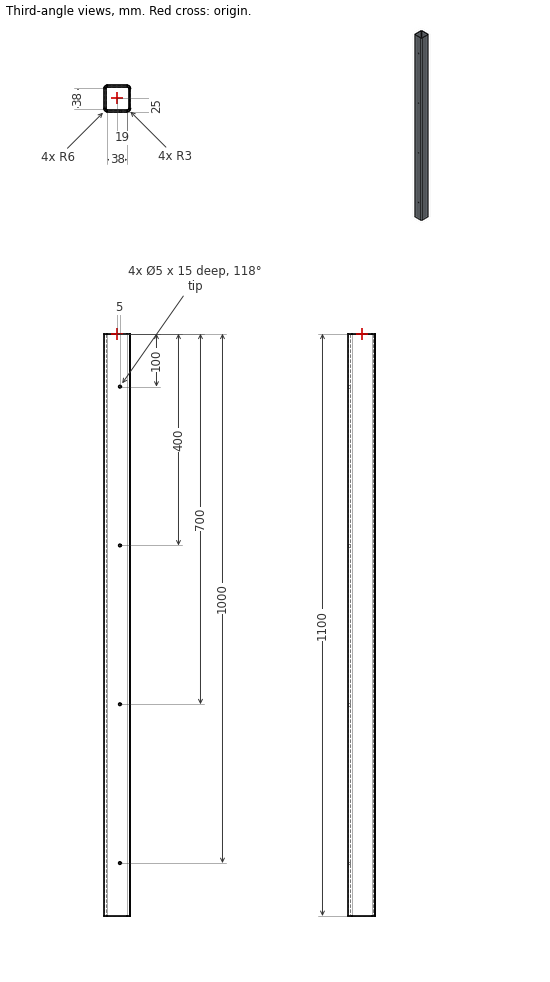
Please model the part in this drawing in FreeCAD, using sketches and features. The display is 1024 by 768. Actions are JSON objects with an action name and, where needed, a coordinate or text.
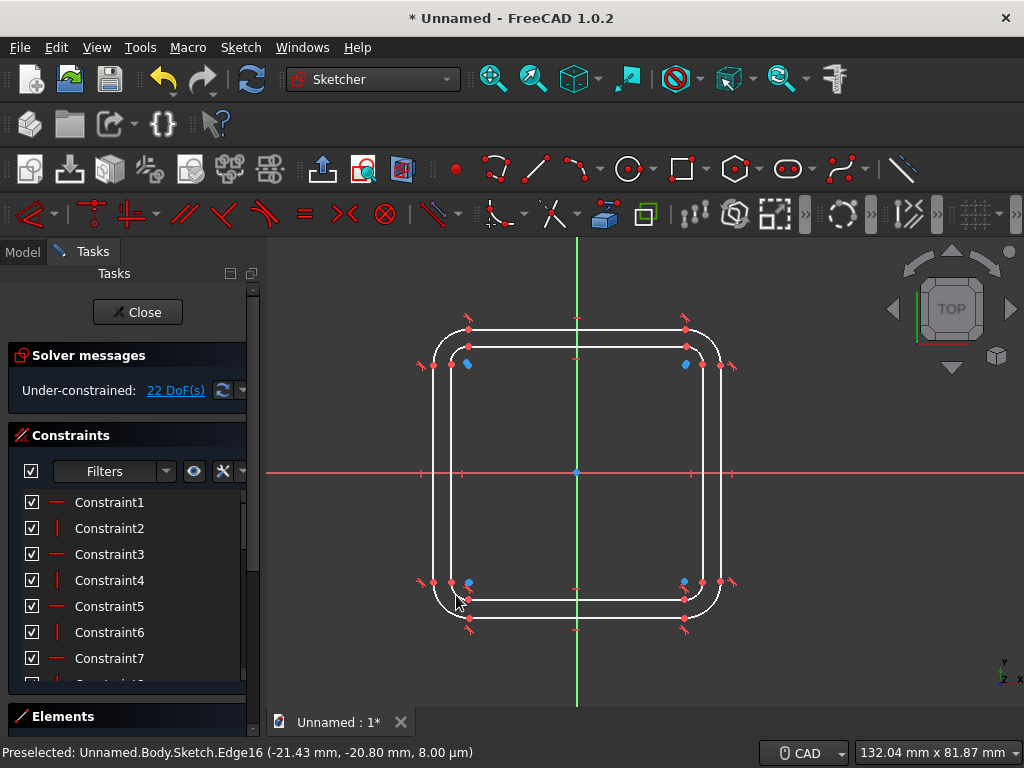
{"action": "left_click", "coordinate": [703, 518]}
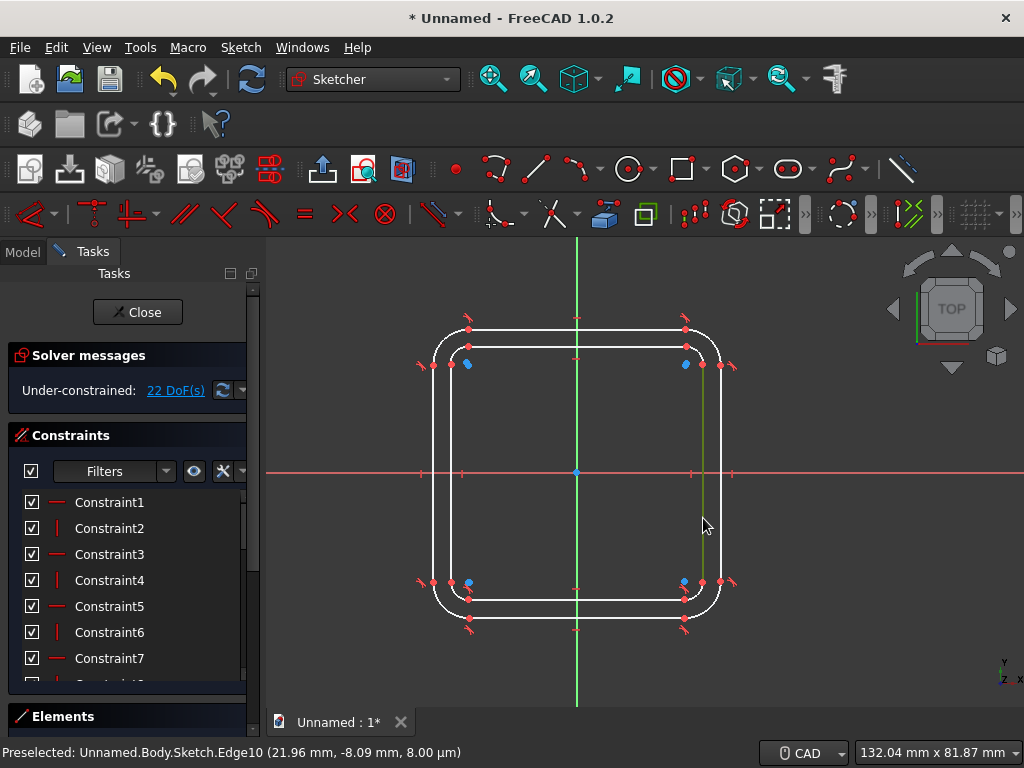
{"action": "left_click", "coordinate": [697, 595]}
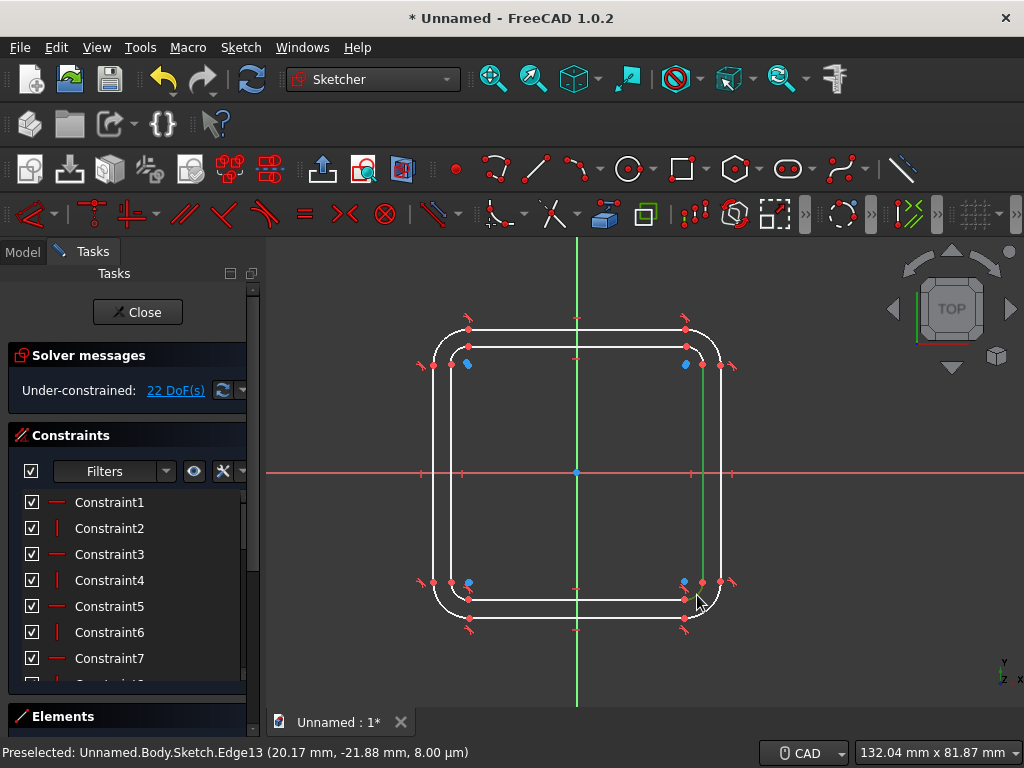
{"action": "key", "text": "t"}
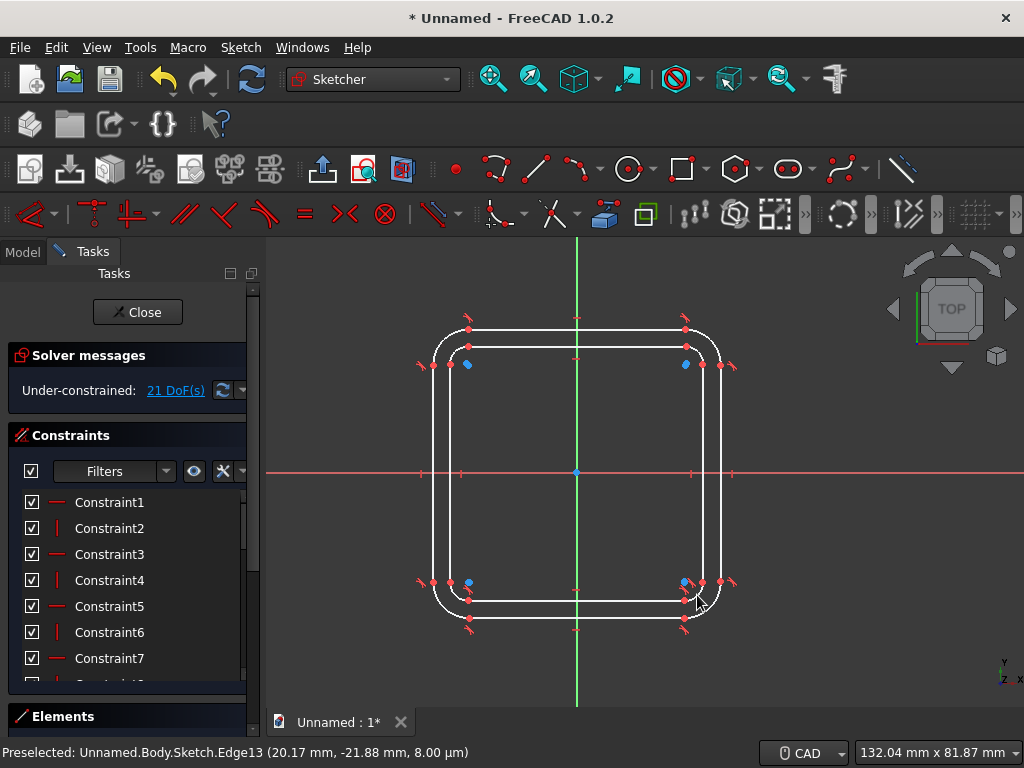
{"action": "left_click", "coordinate": [703, 517]}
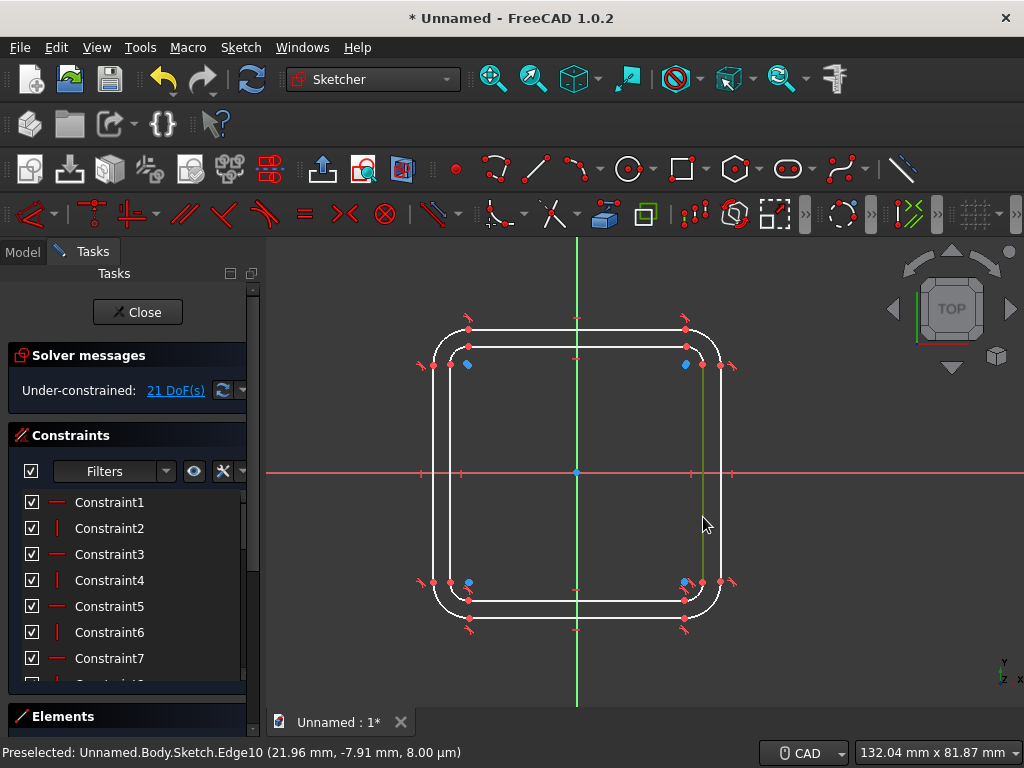
{"action": "left_click", "coordinate": [699, 352]}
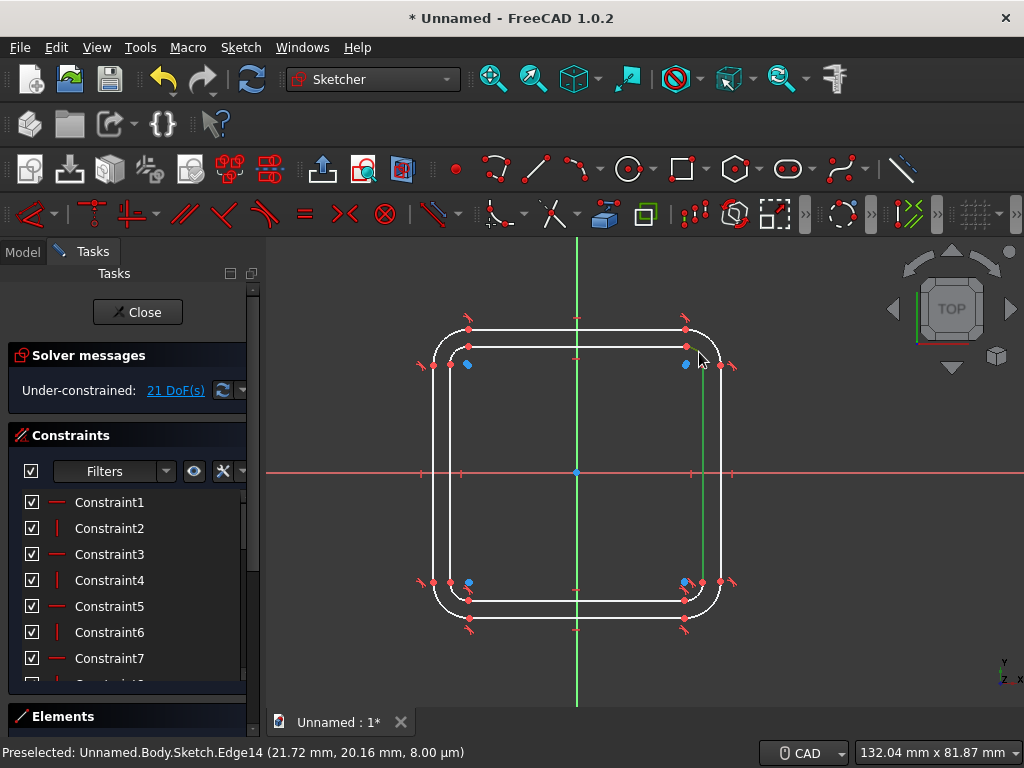
{"action": "key", "text": "t"}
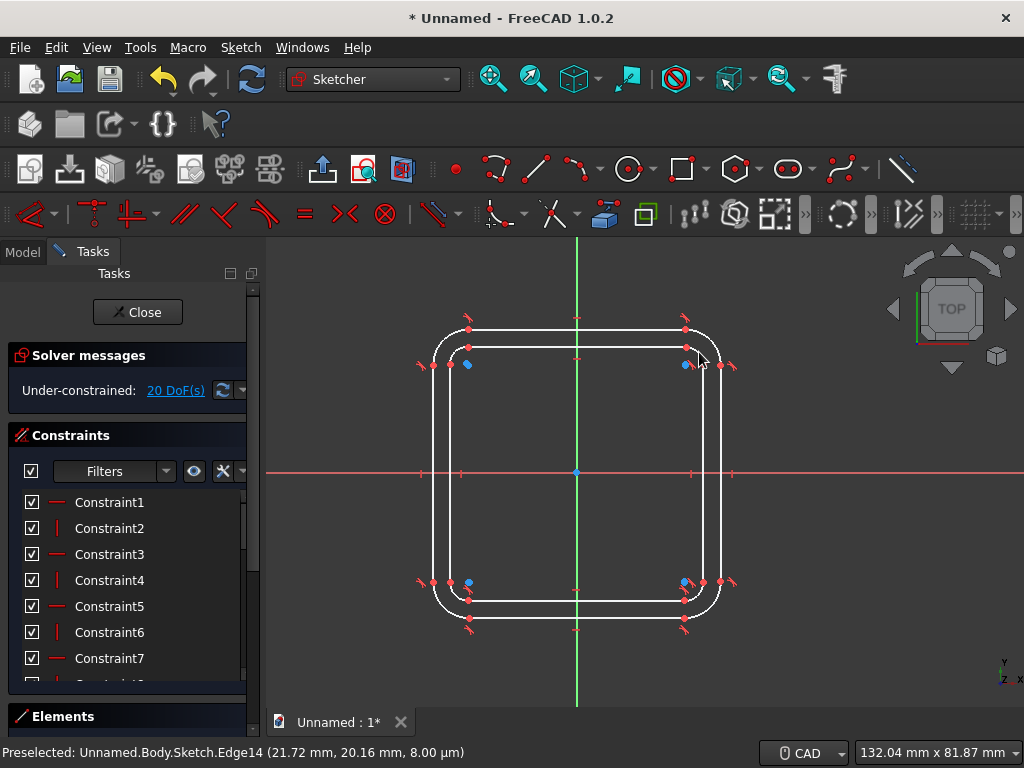
{"action": "left_click", "coordinate": [621, 347]}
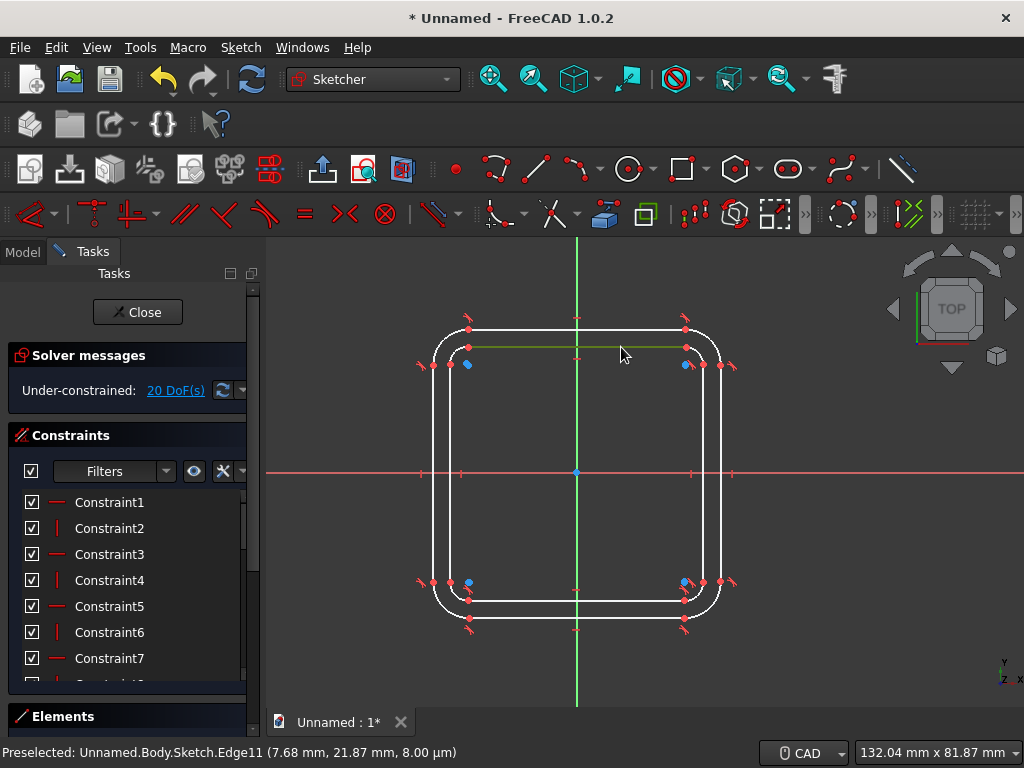
{"action": "left_click", "coordinate": [698, 353]}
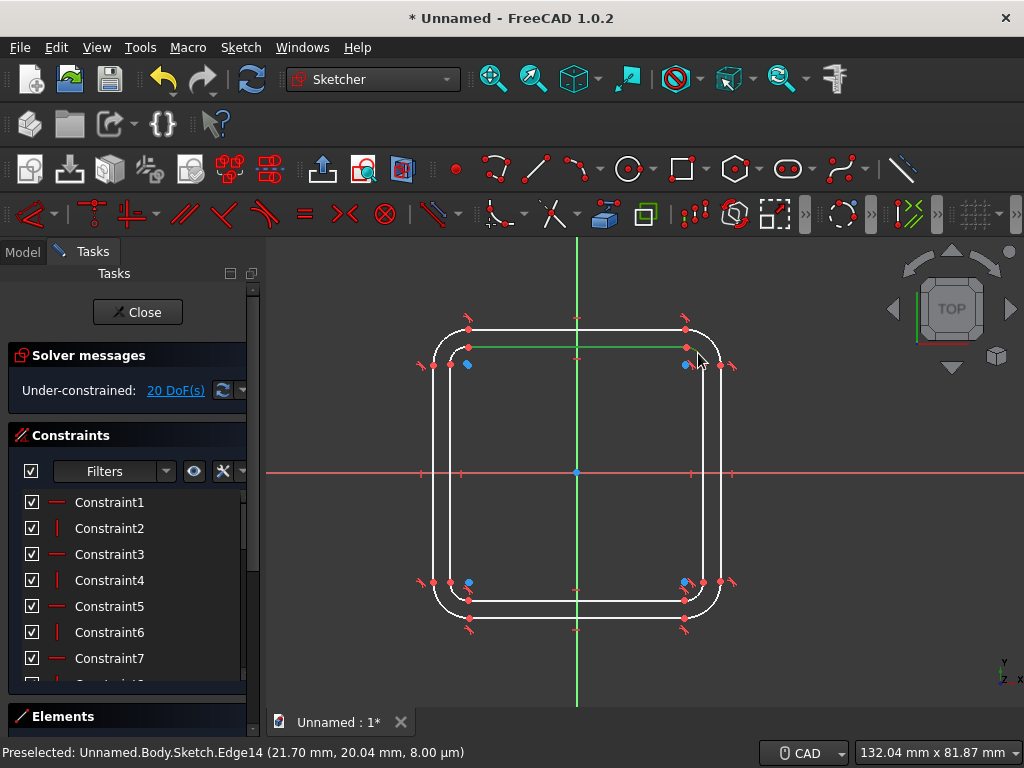
{"action": "key", "text": "t"}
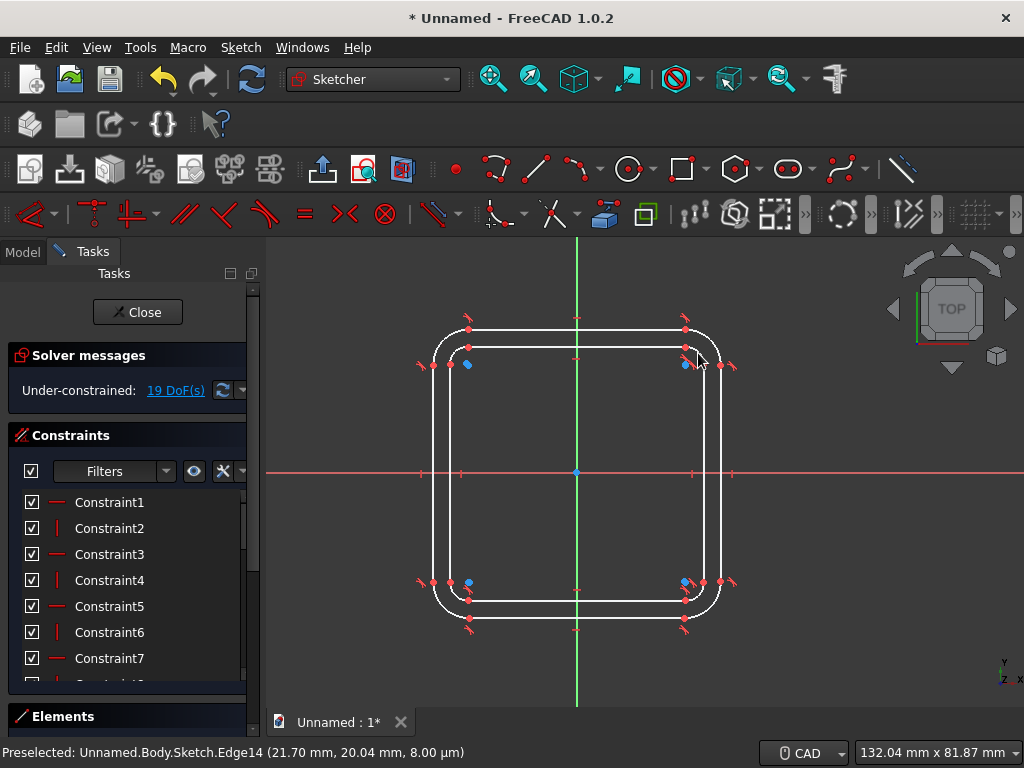
{"action": "left_click", "coordinate": [621, 347]}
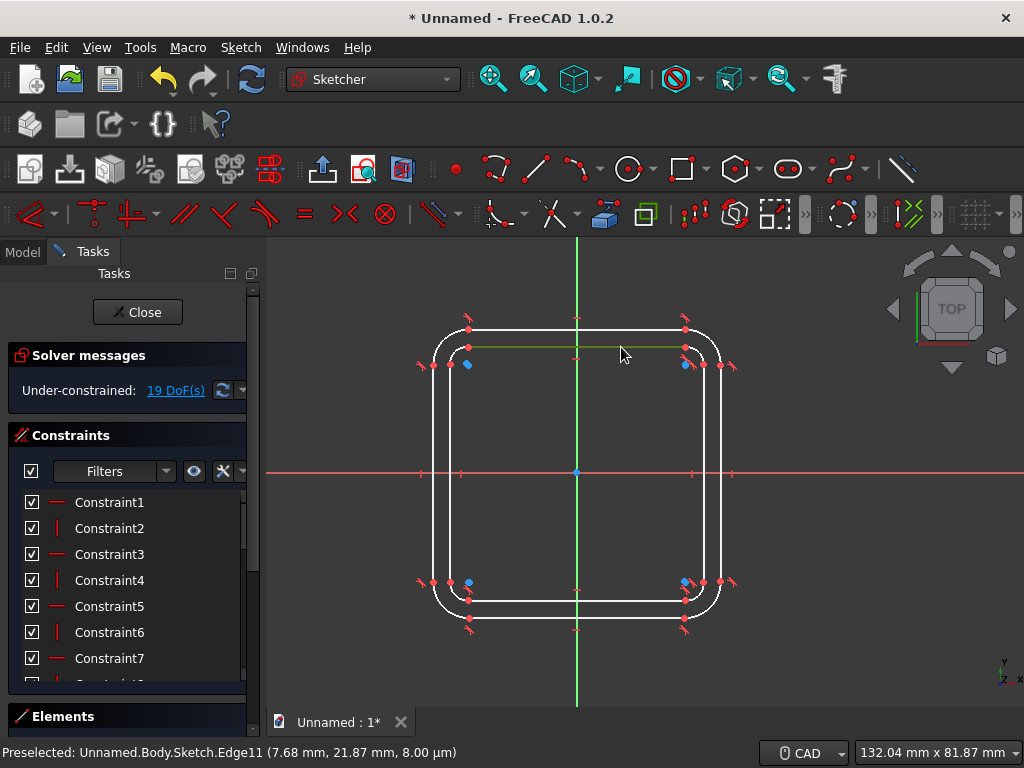
{"action": "left_click", "coordinate": [455, 352]}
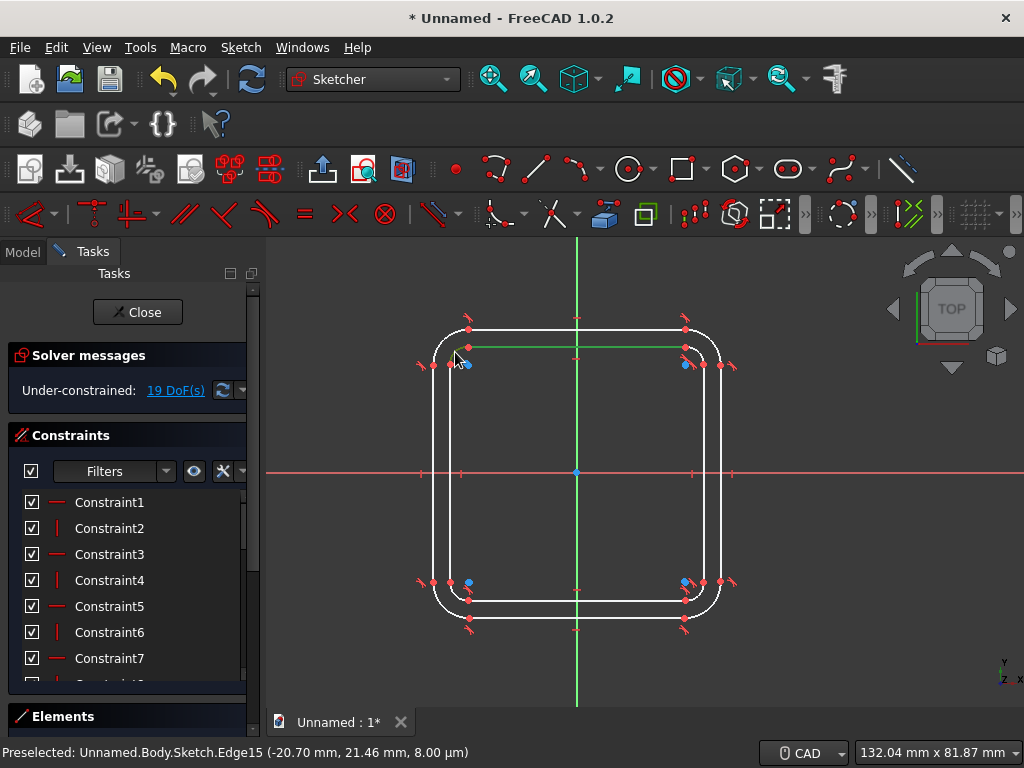
{"action": "key", "text": "t"}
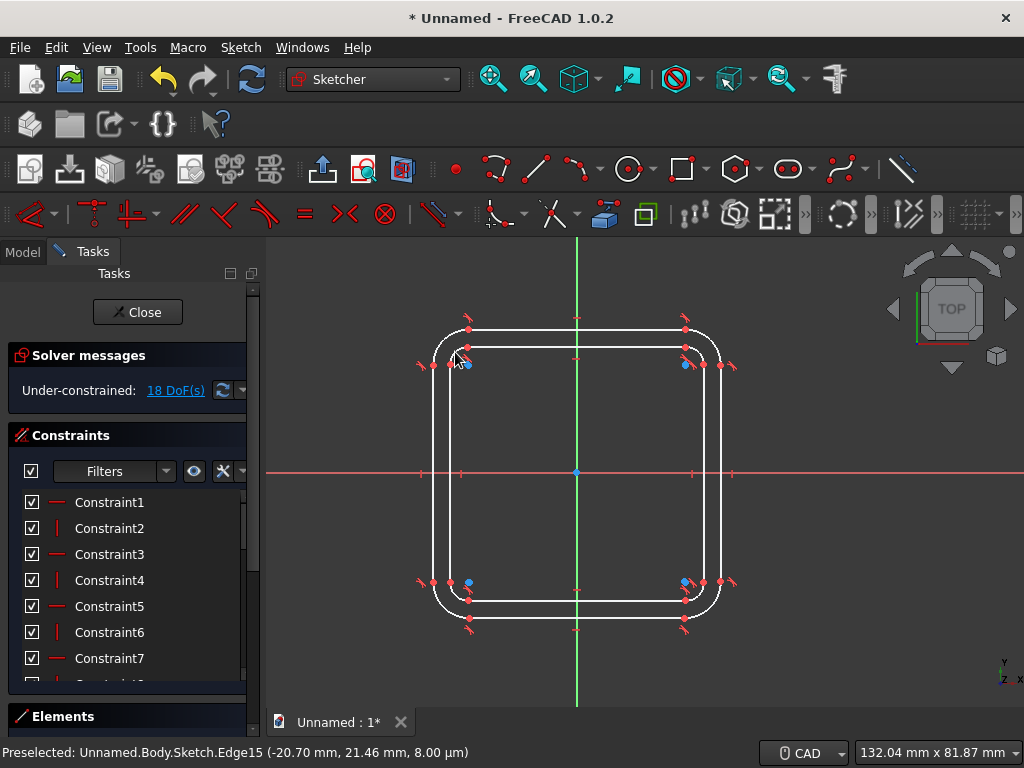
{"action": "left_click", "coordinate": [450, 430]}